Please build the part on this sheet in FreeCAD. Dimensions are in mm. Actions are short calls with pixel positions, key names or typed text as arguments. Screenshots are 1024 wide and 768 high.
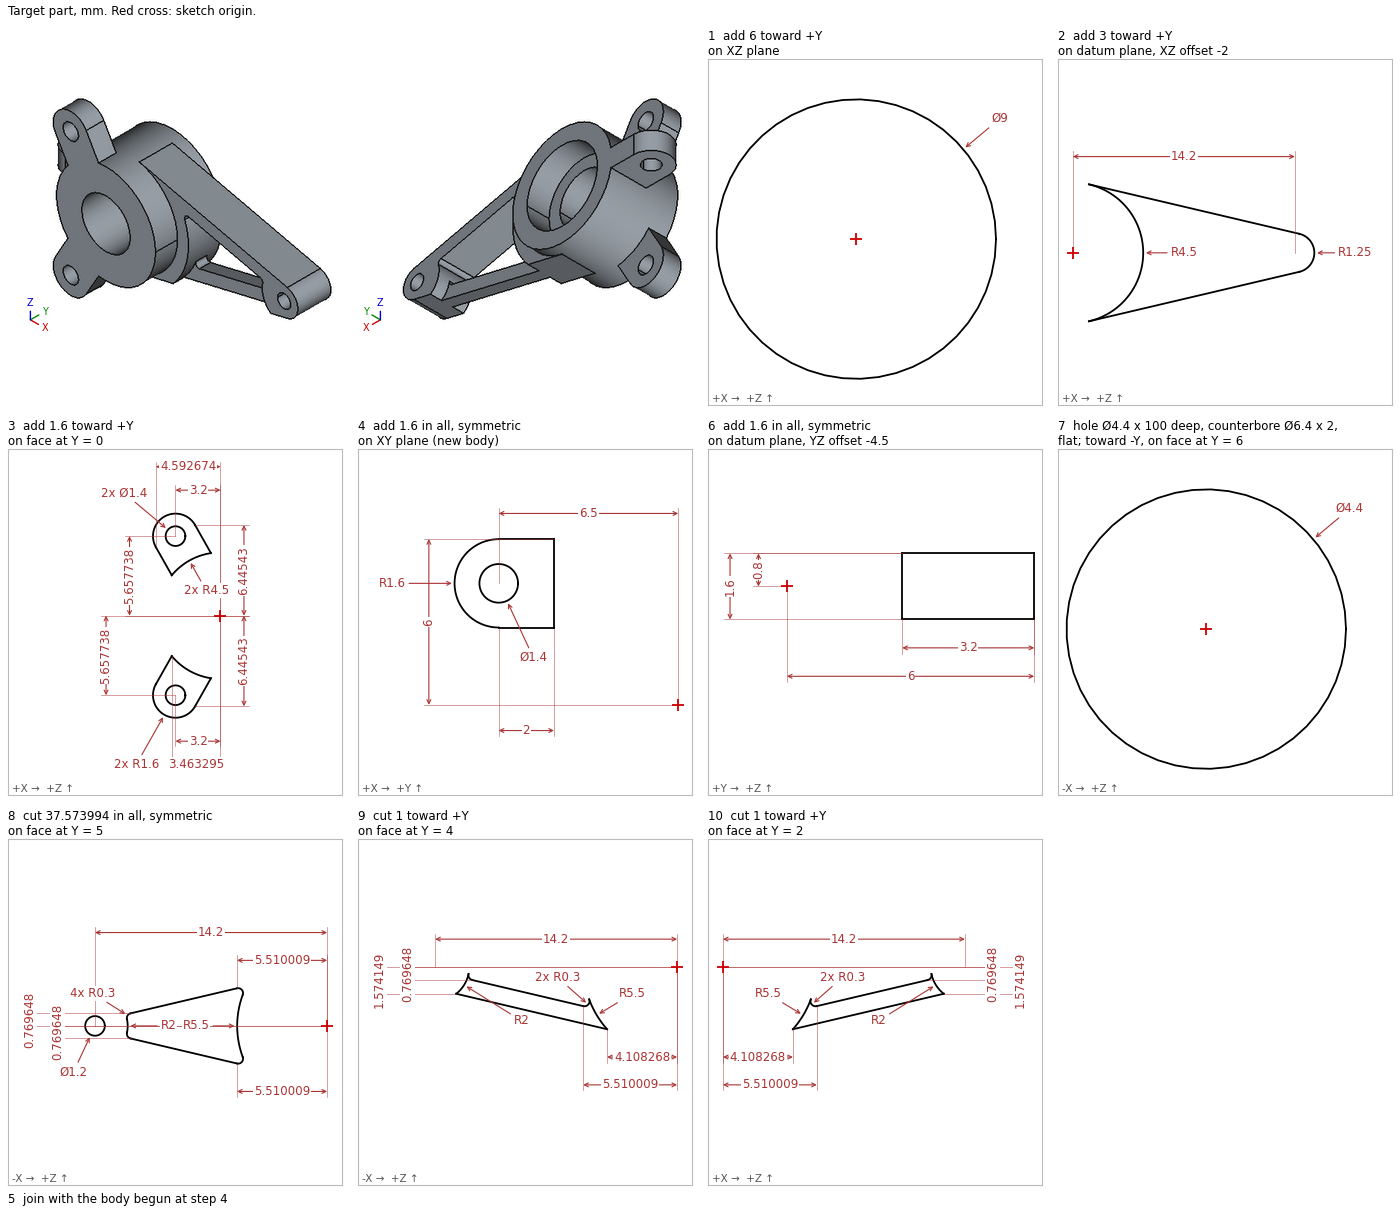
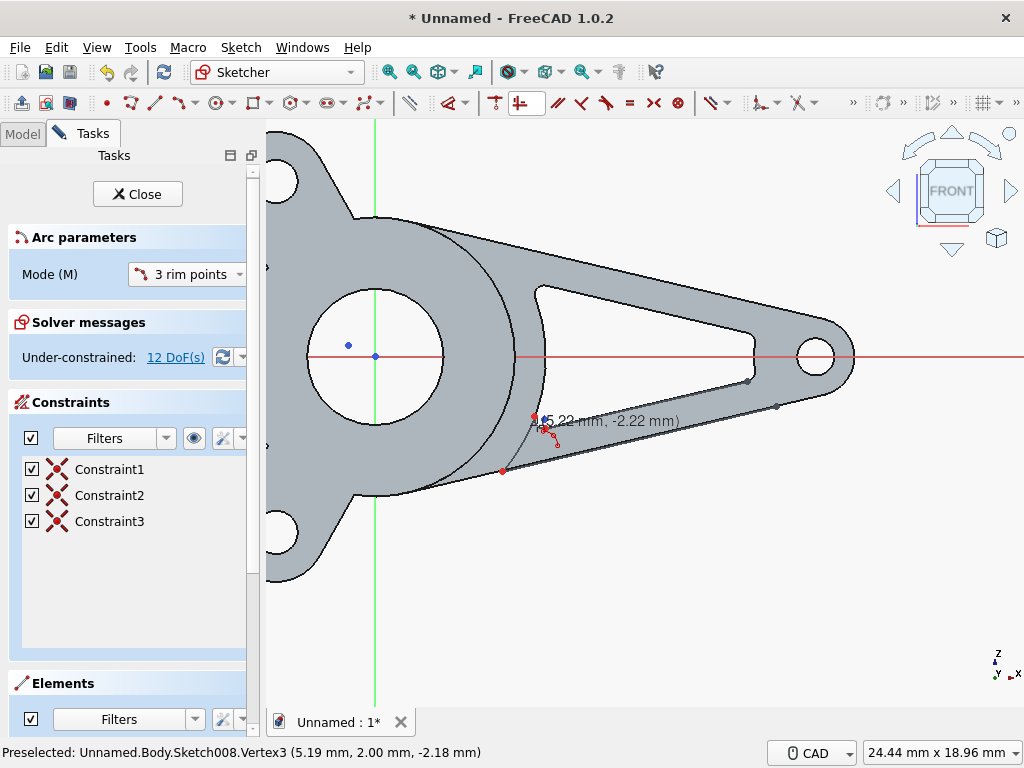
click(748, 382)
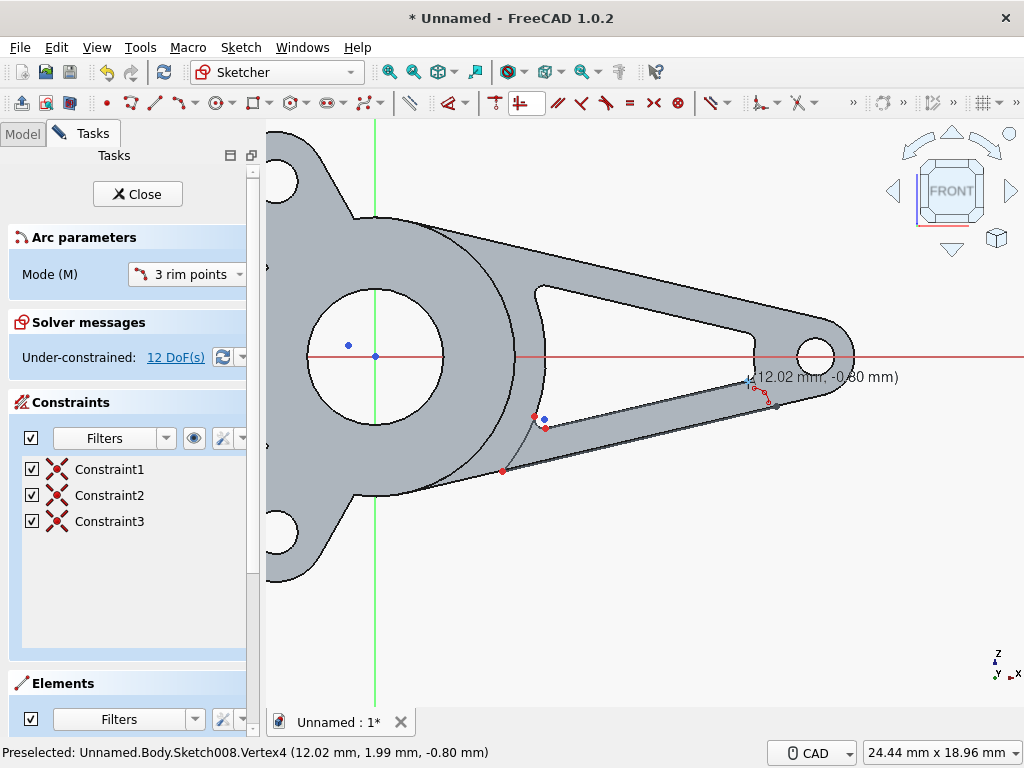
scroll(755, 370, up, 2)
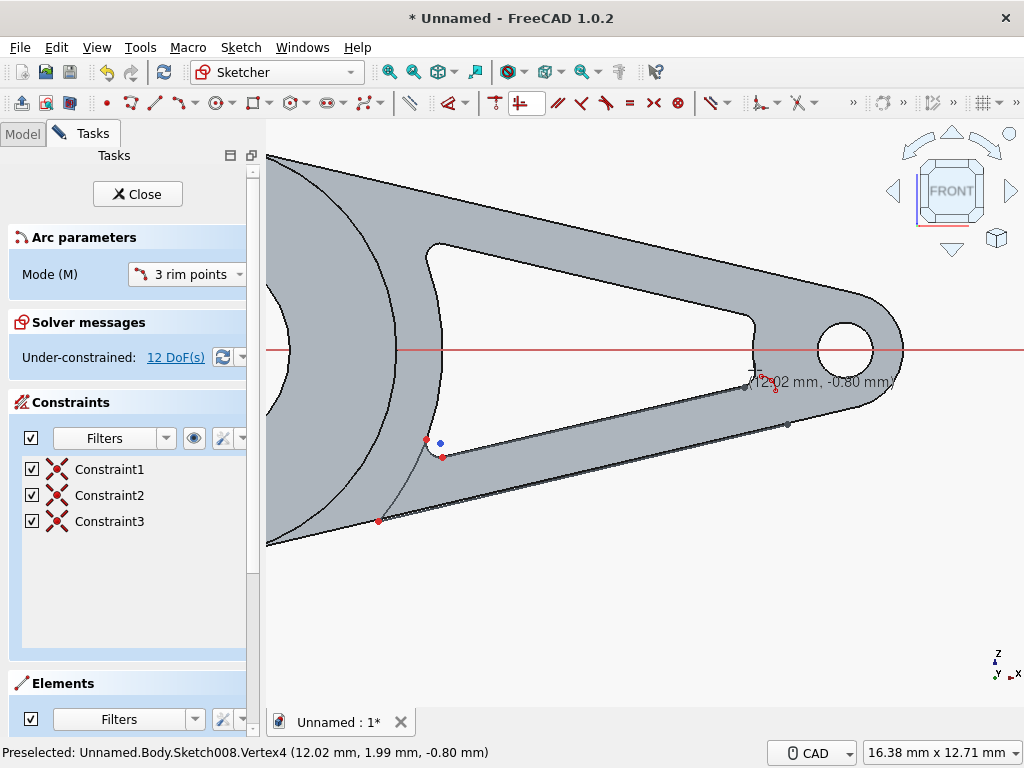
click(755, 370)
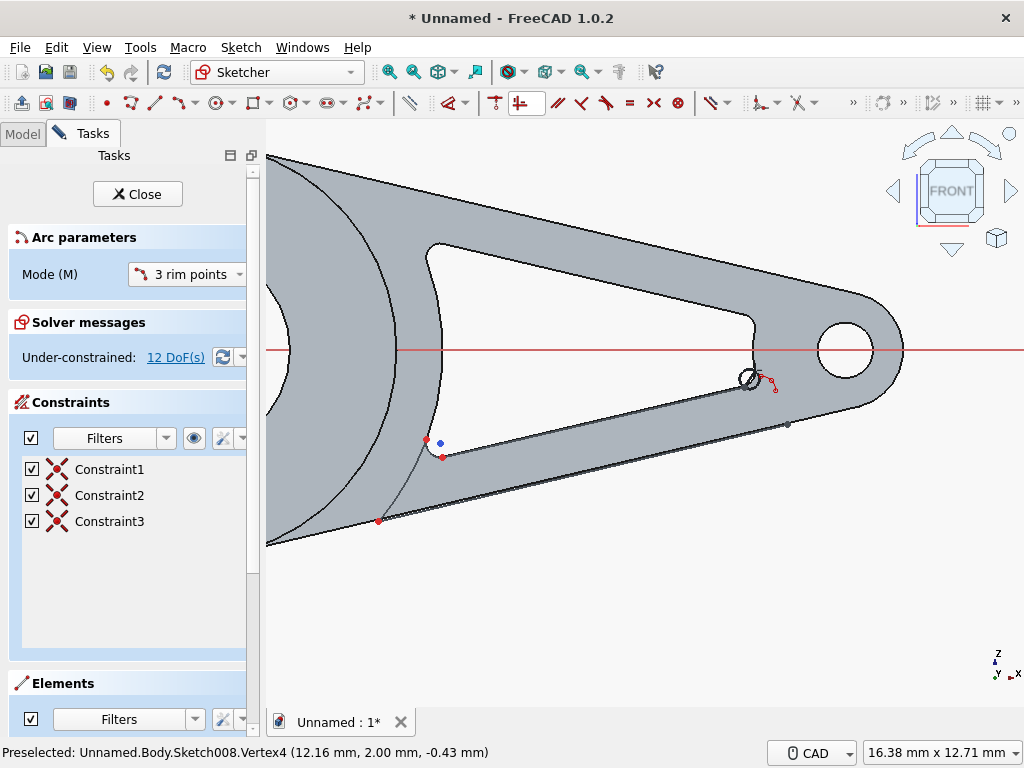
scroll(753, 380, up, 7)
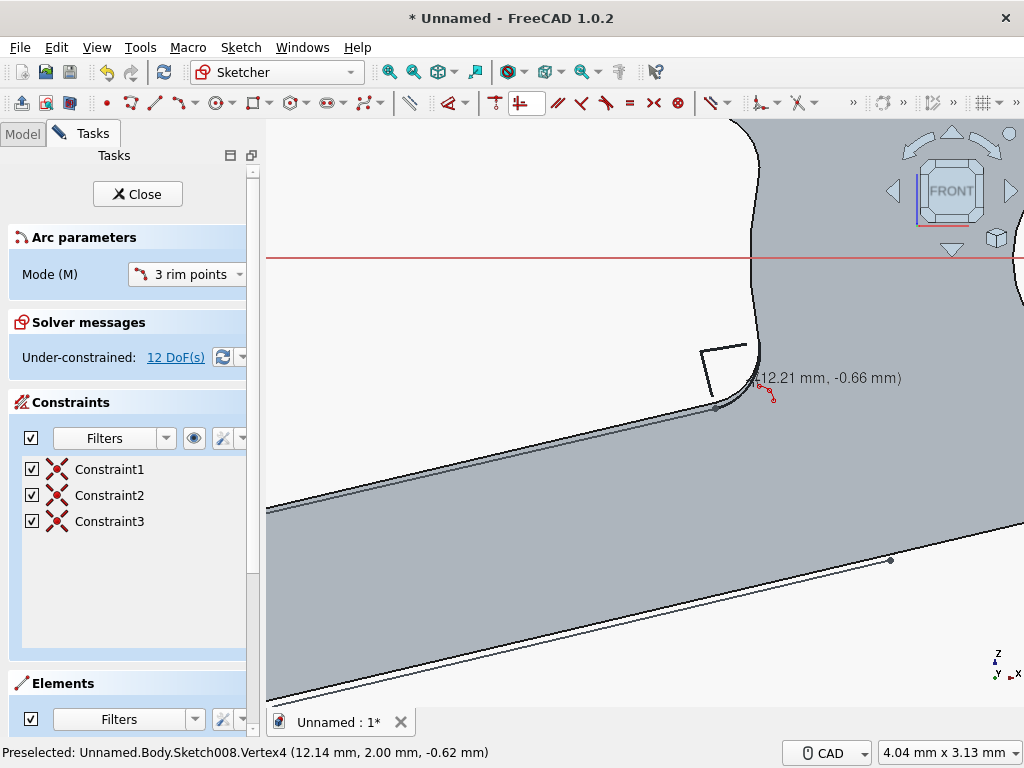
click(751, 378)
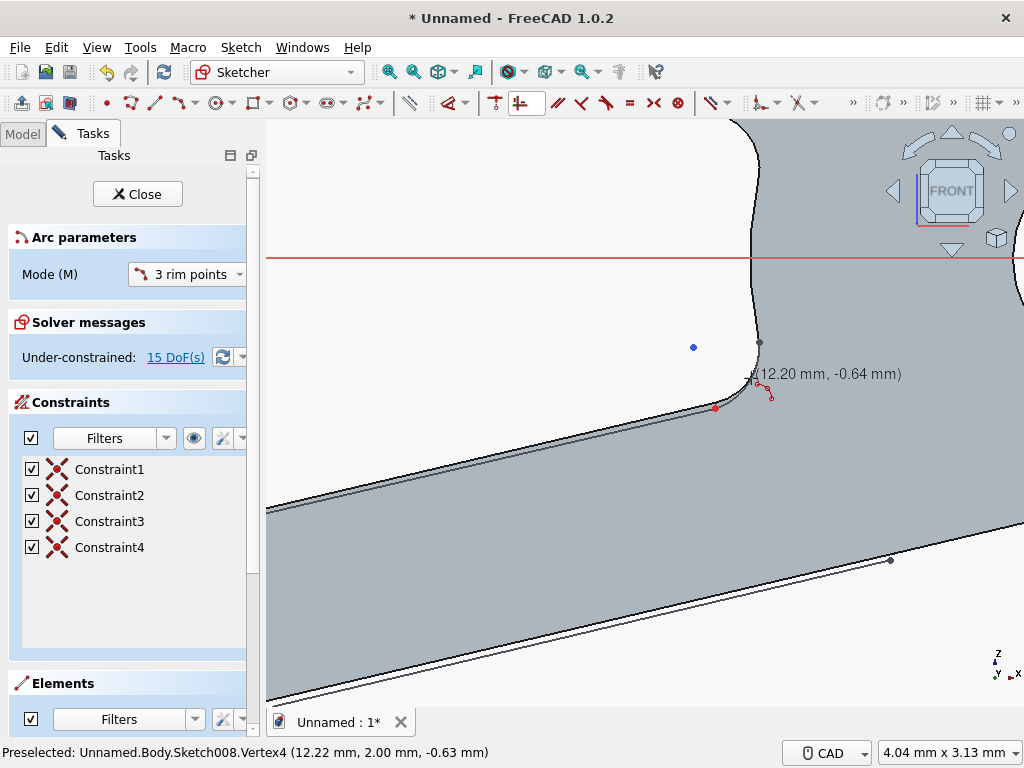
scroll(755, 376, down, 9)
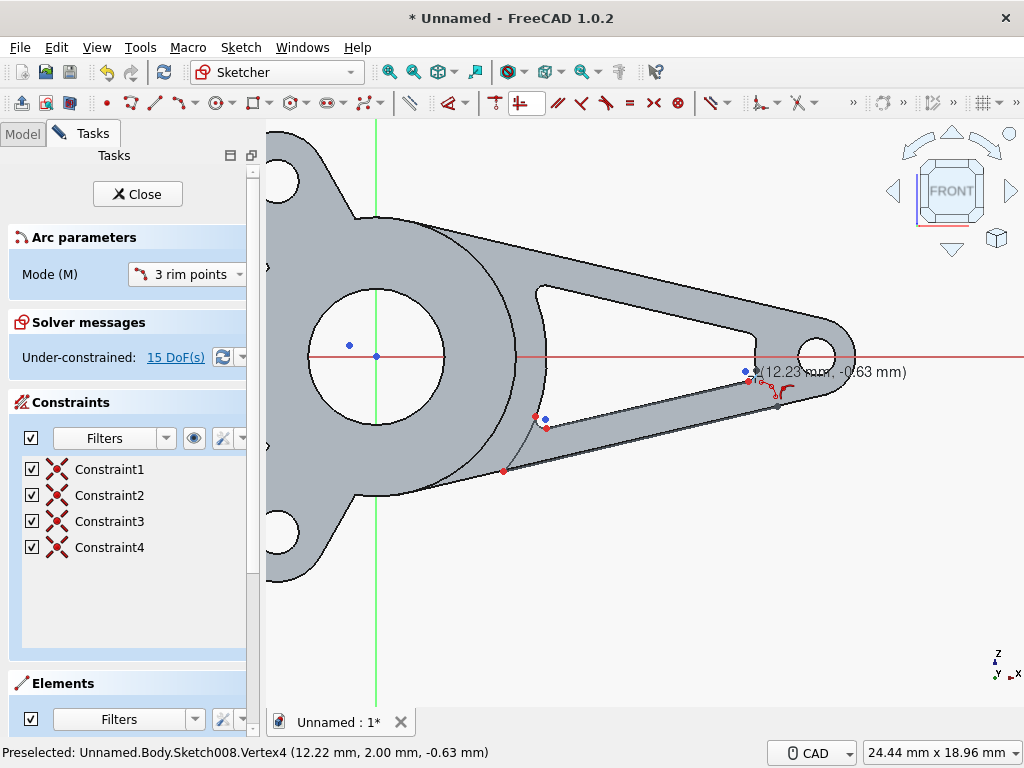
scroll(756, 370, up, 3)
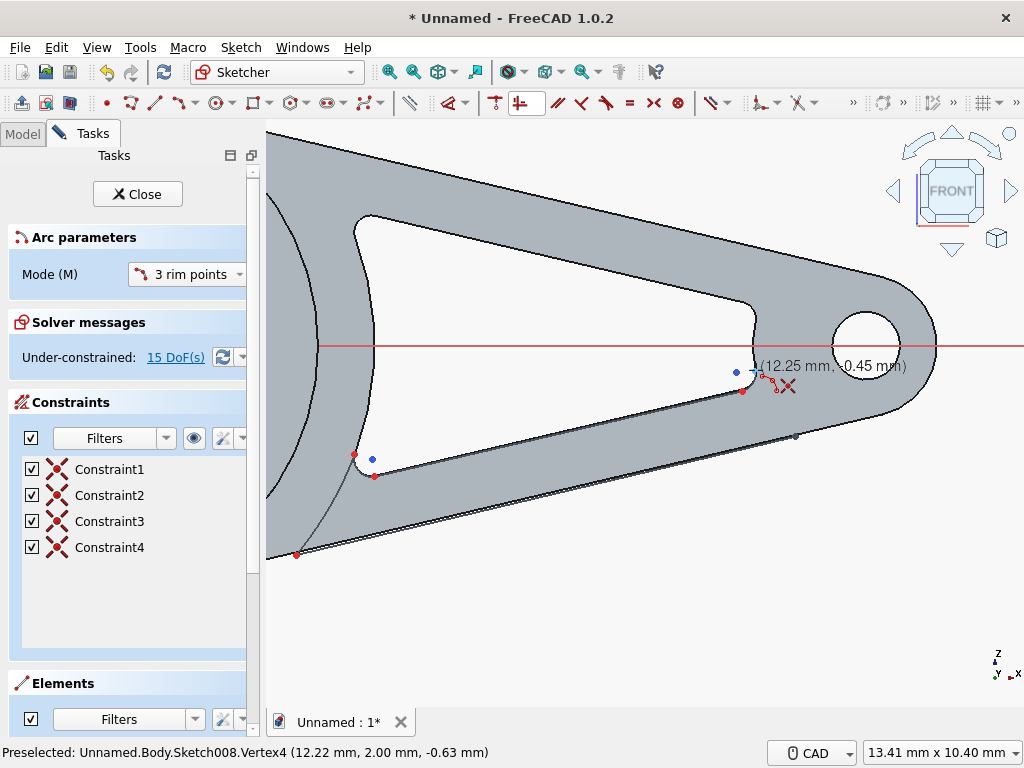
click(756, 371)
click(796, 437)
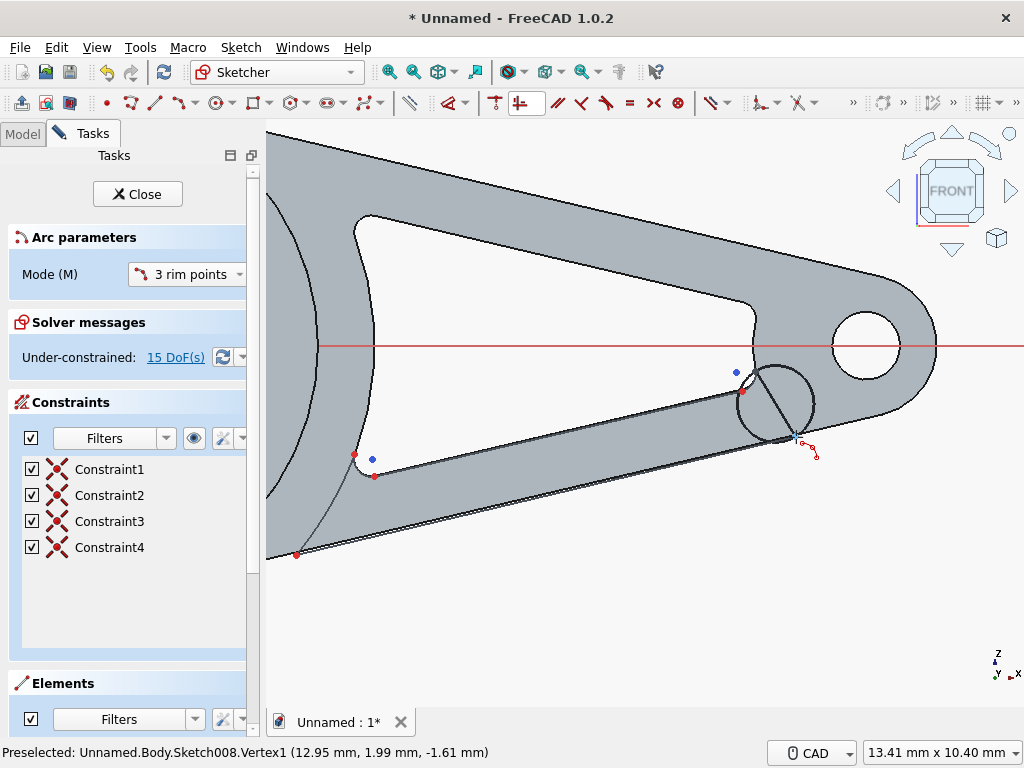
scroll(770, 406, up, 5)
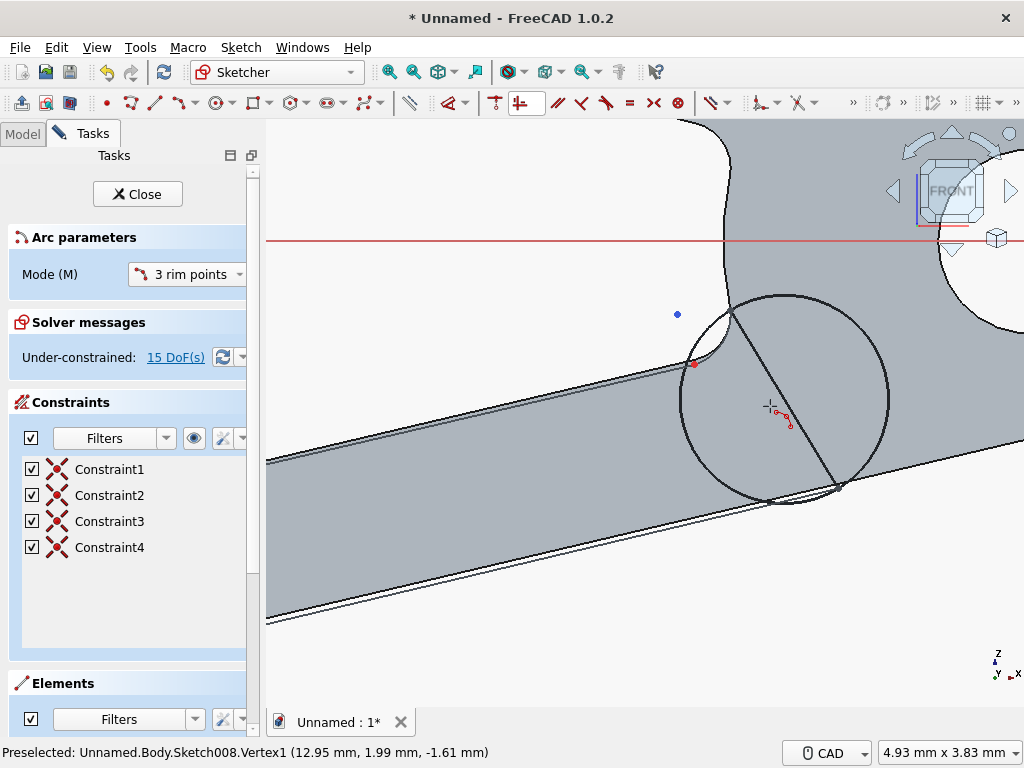
click(770, 404)
key(Escape)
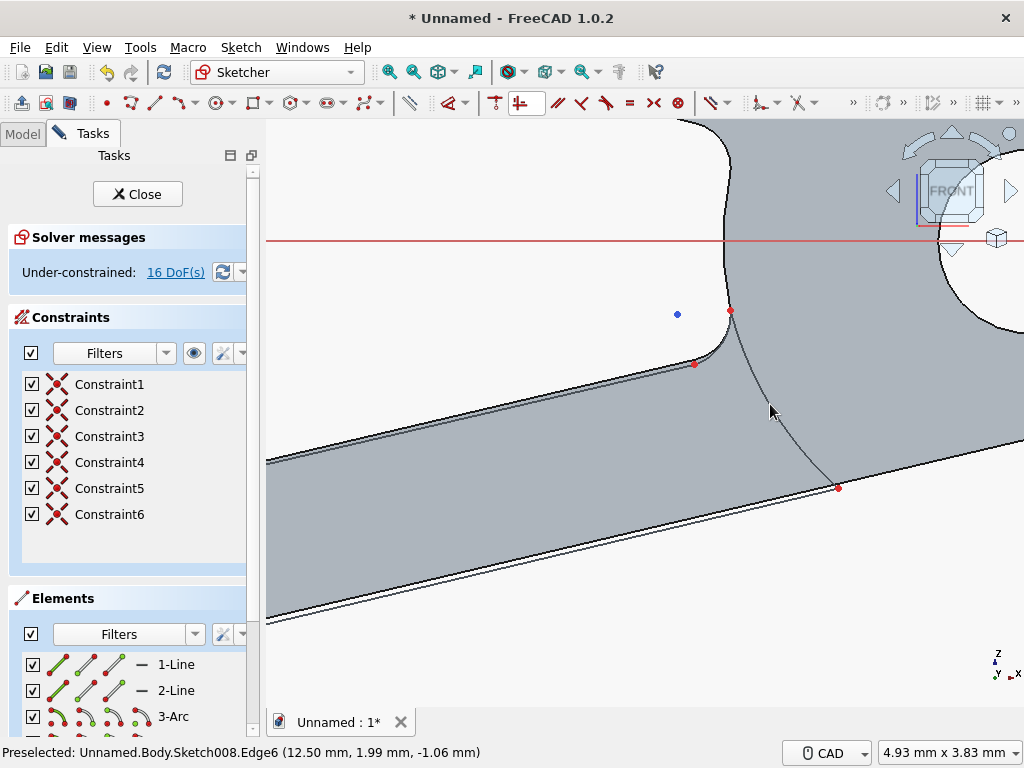
scroll(762, 385, down, 8)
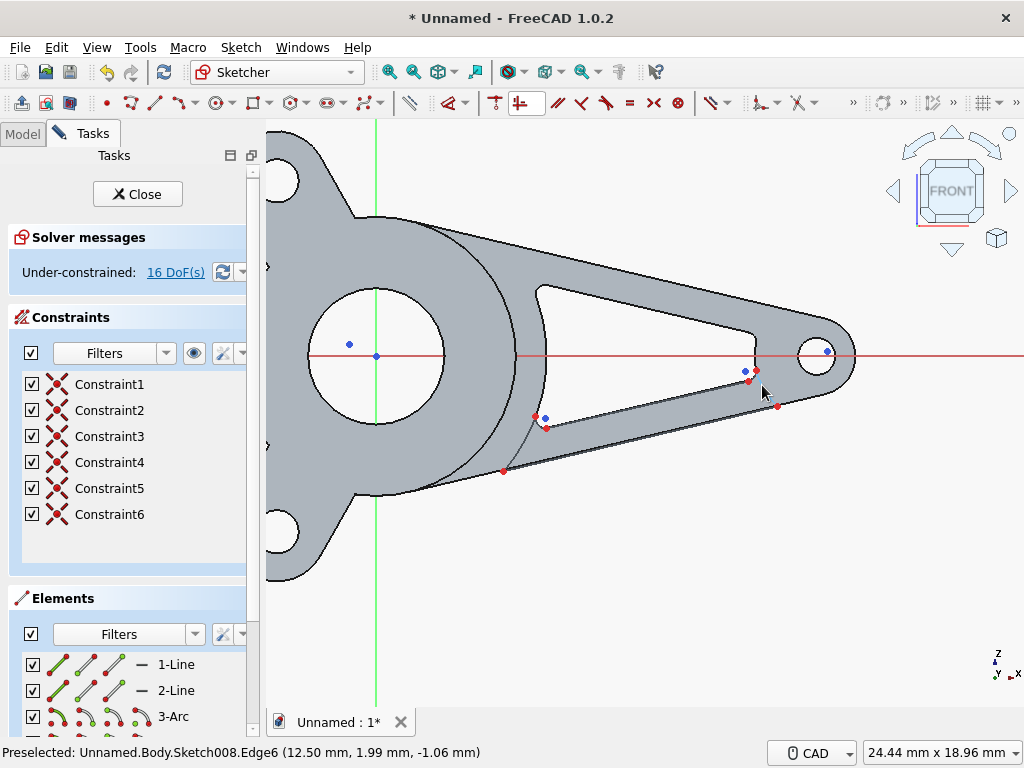
click(688, 395)